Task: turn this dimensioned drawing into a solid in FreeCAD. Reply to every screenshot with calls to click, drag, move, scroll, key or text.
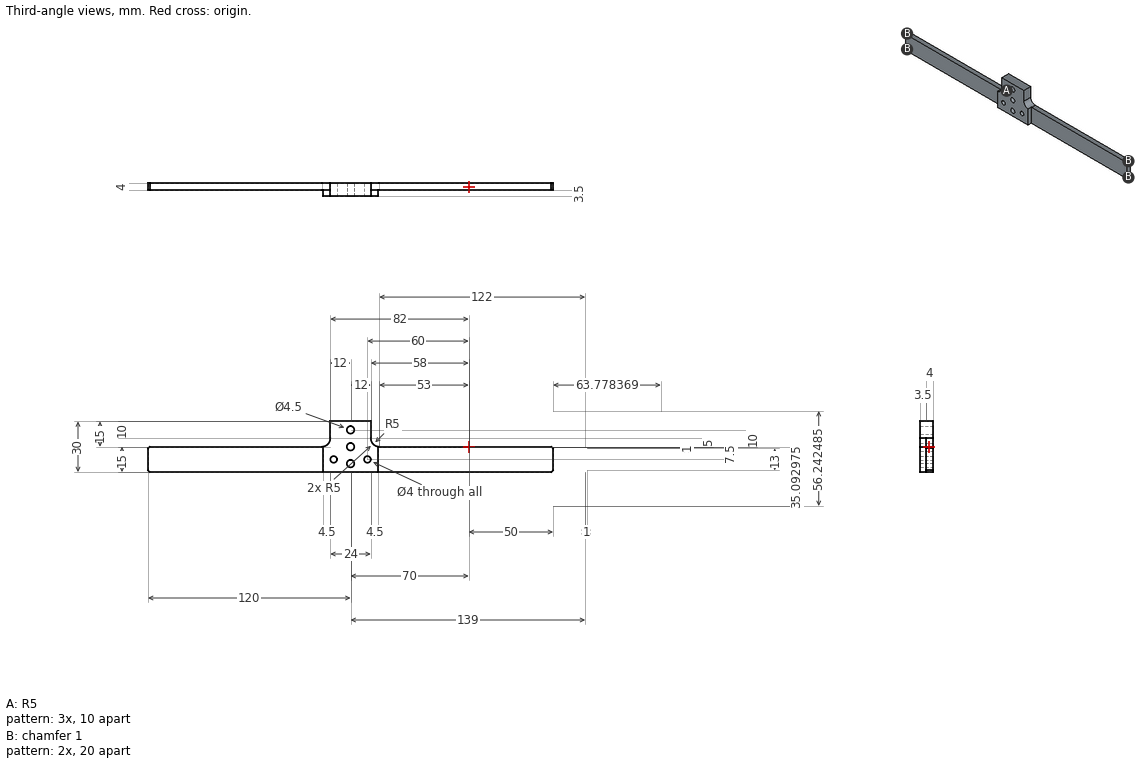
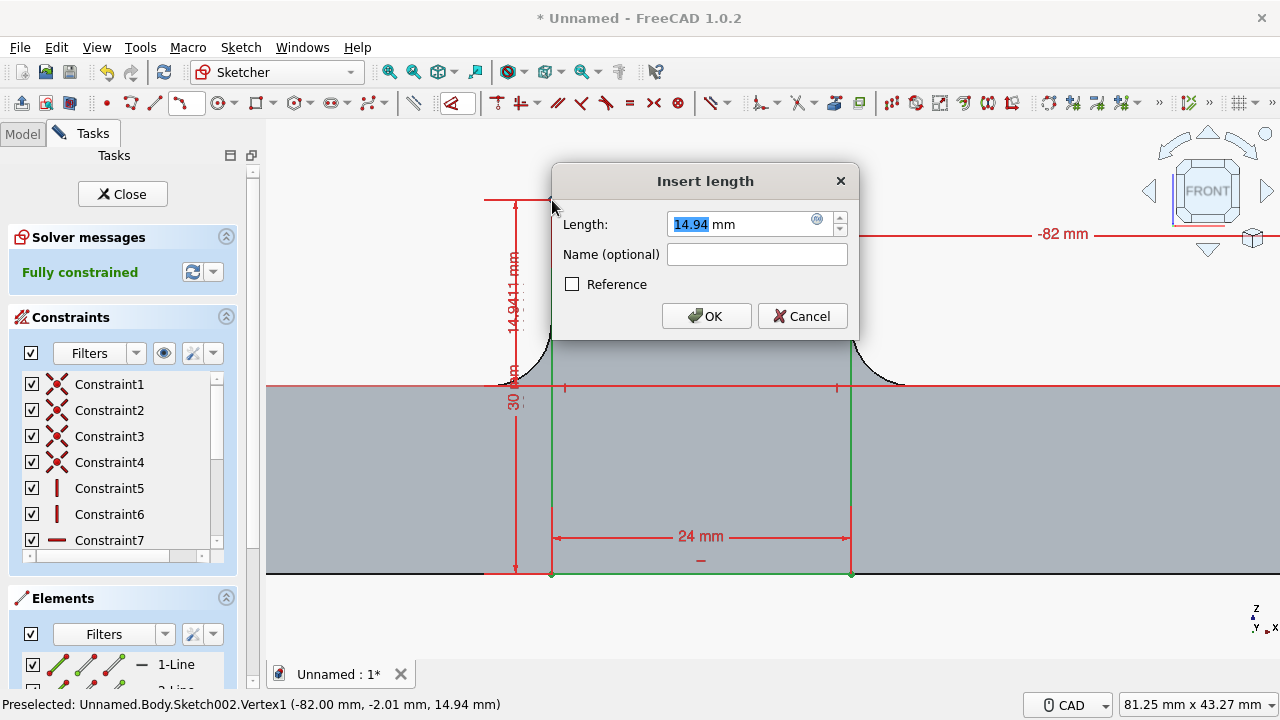
text(15)
key(Return)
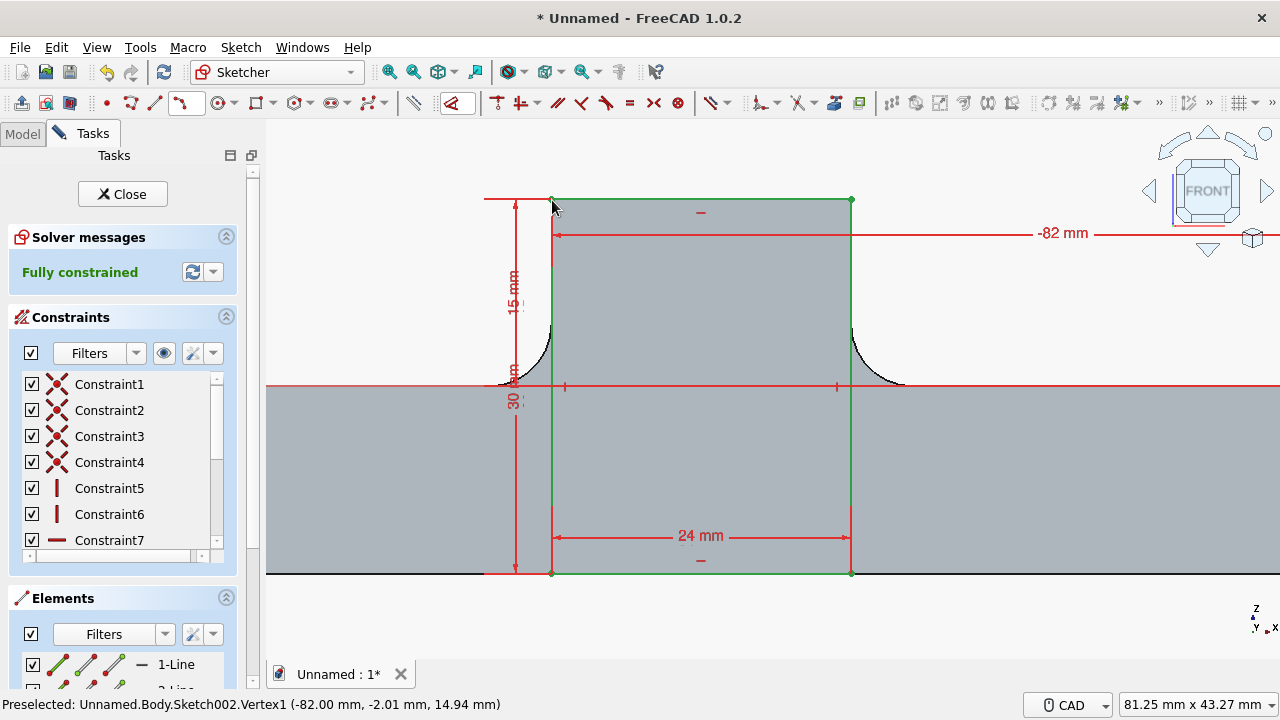
click(123, 194)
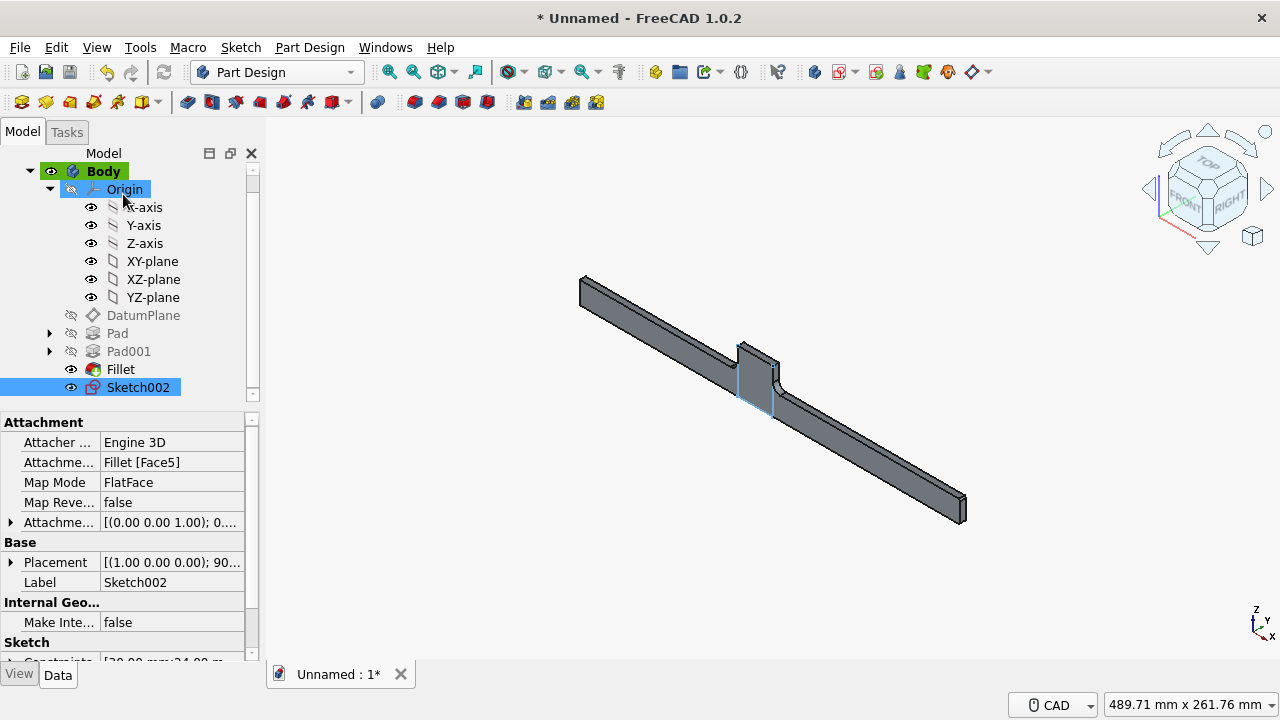
click(22, 102)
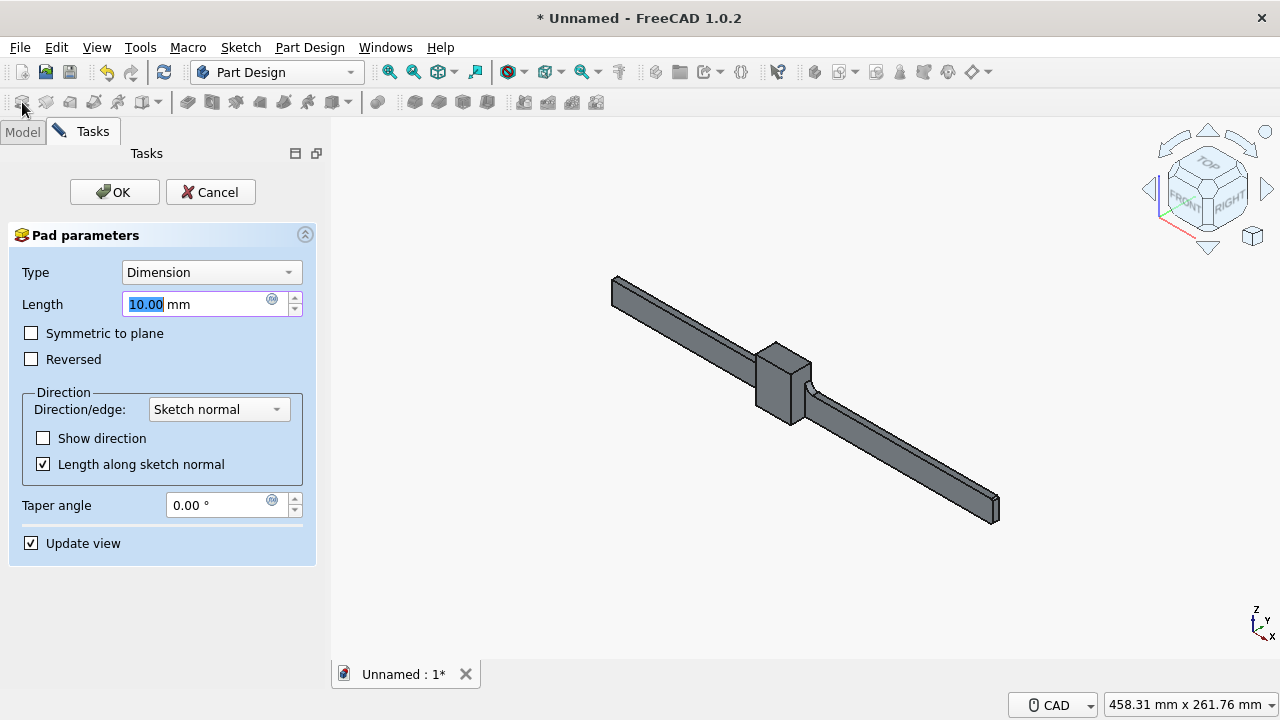
text(3.5)
key(Tab)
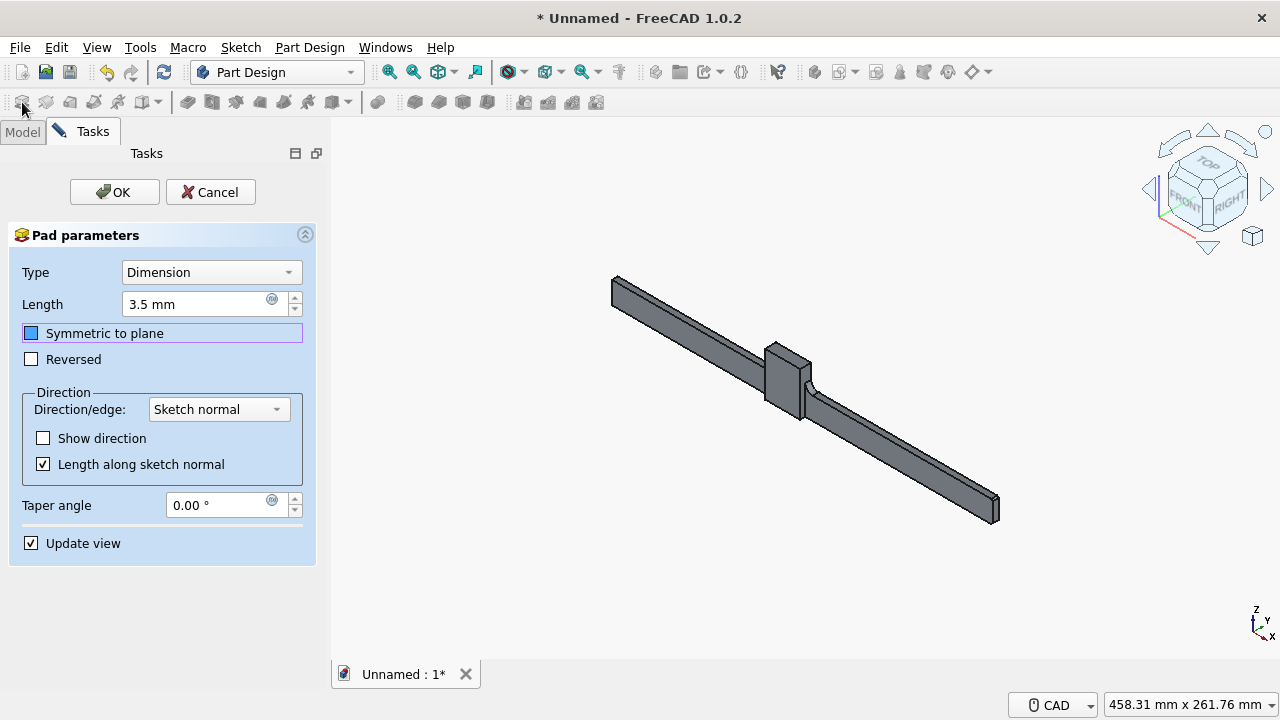
click(115, 192)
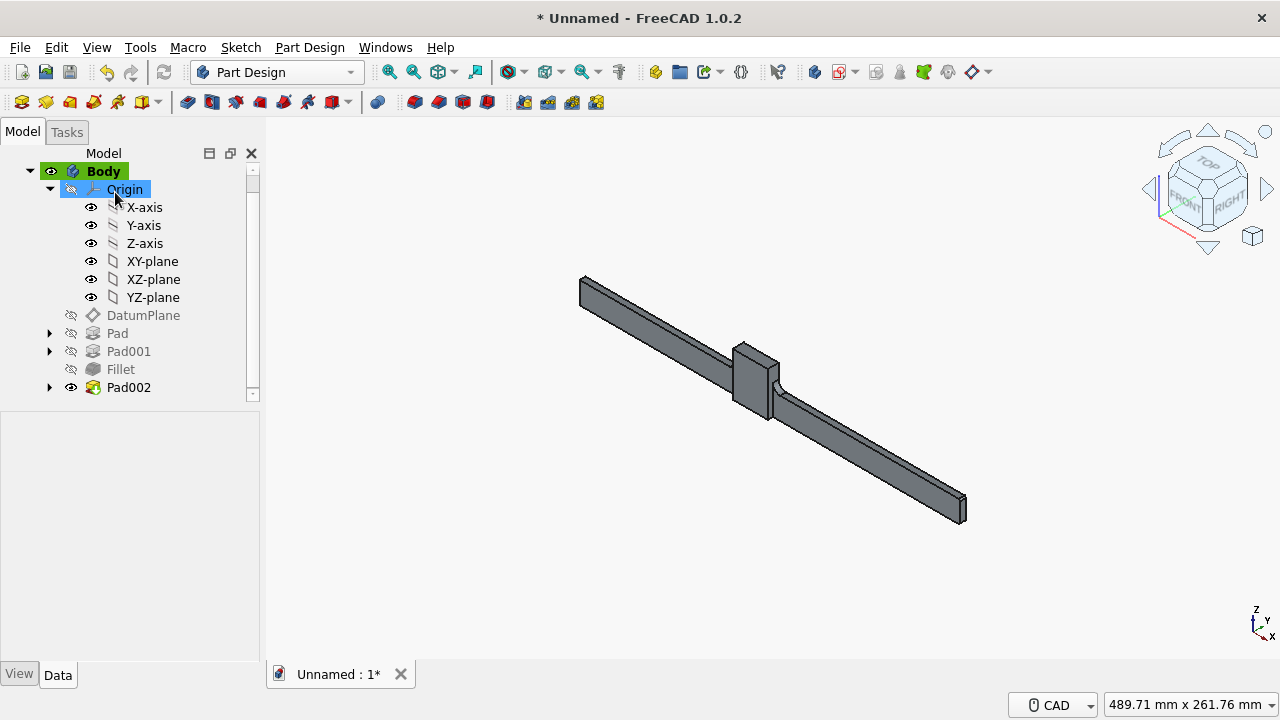
key(4)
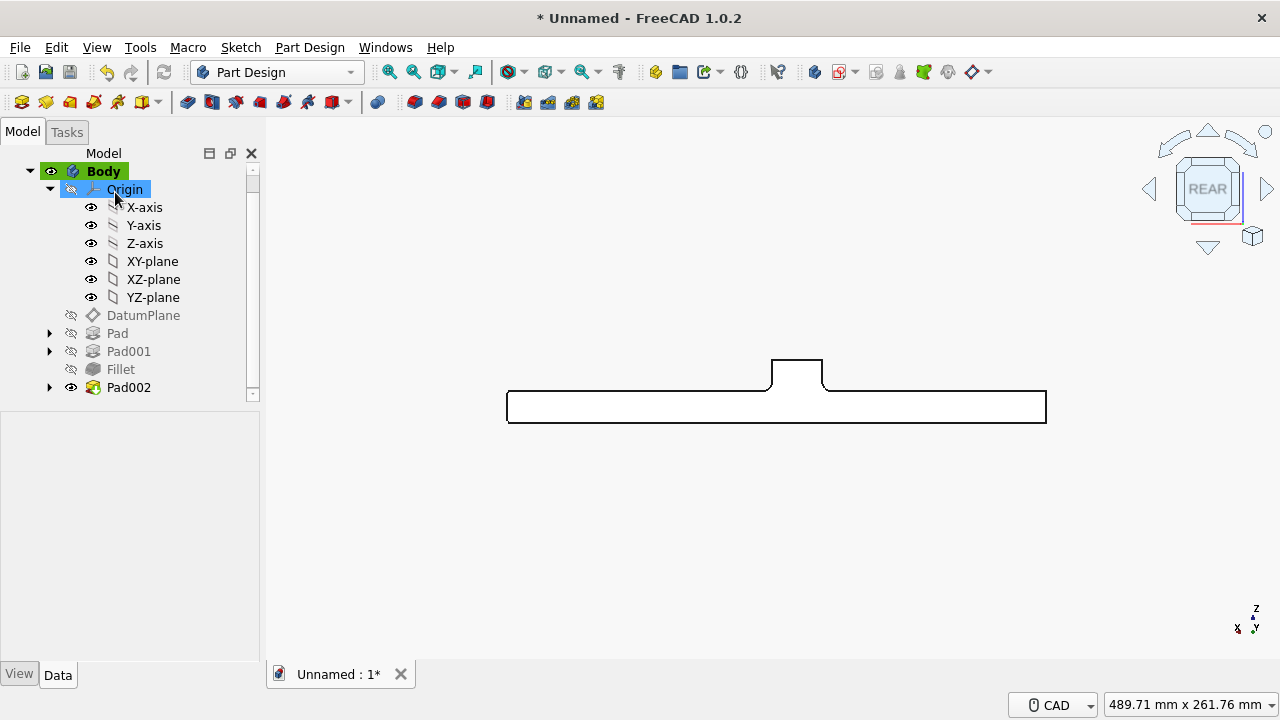
click(776, 399)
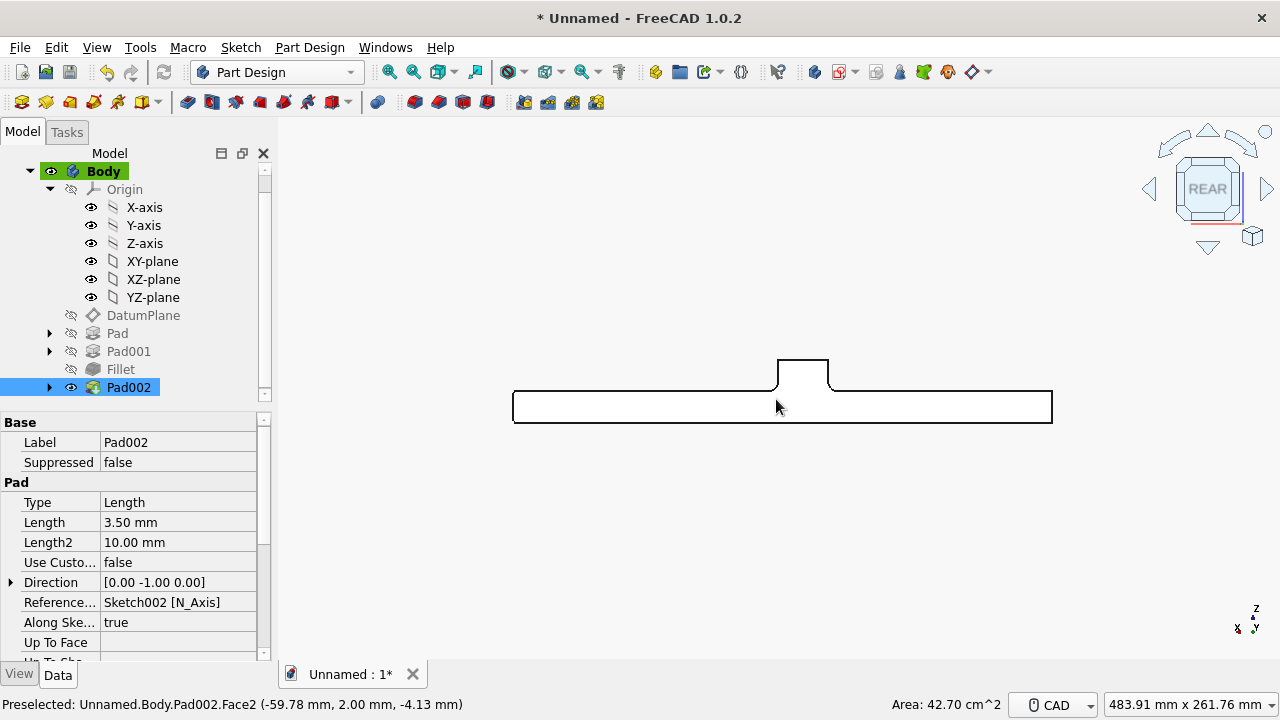
click(840, 72)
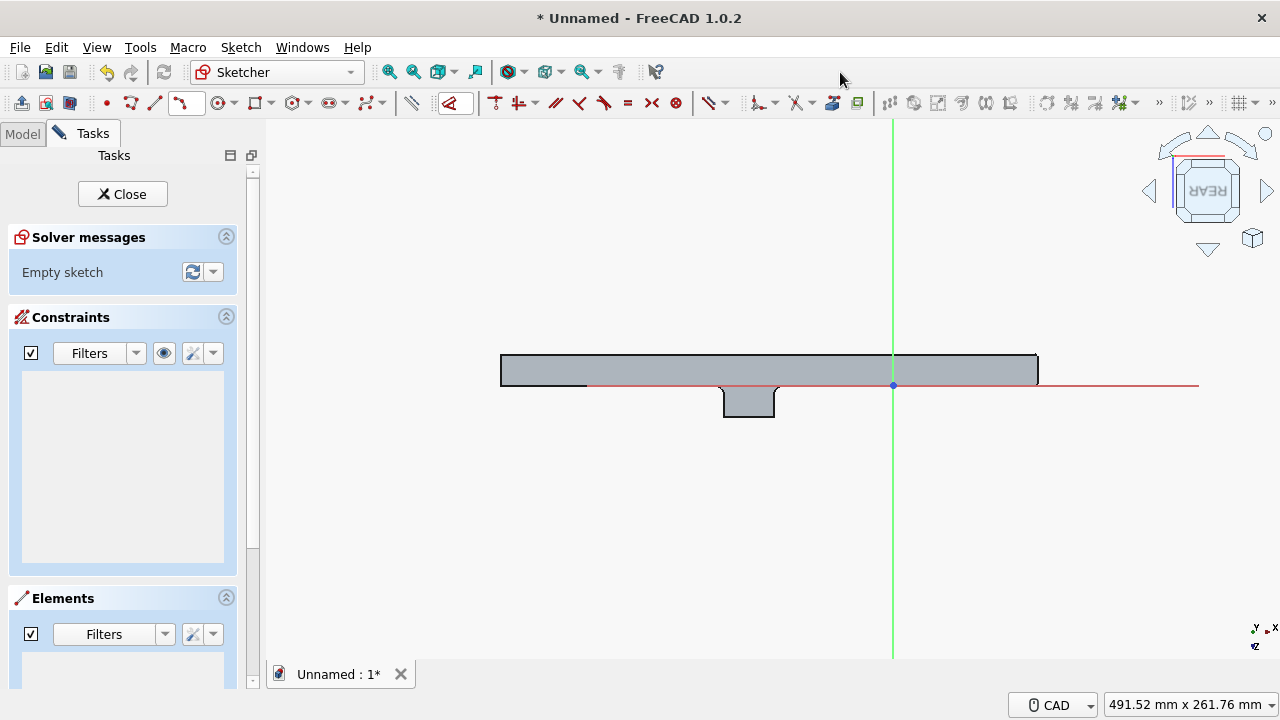
scroll(751, 407, up, 15)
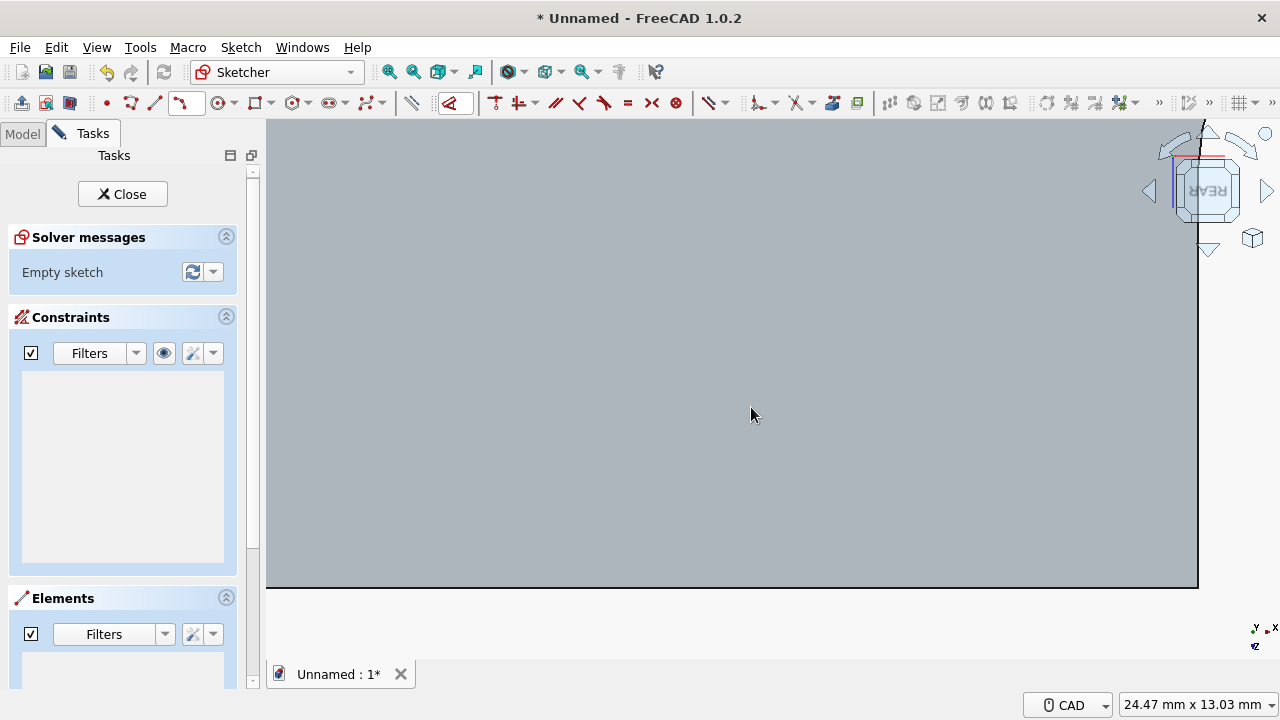
scroll(695, 370, up, 3)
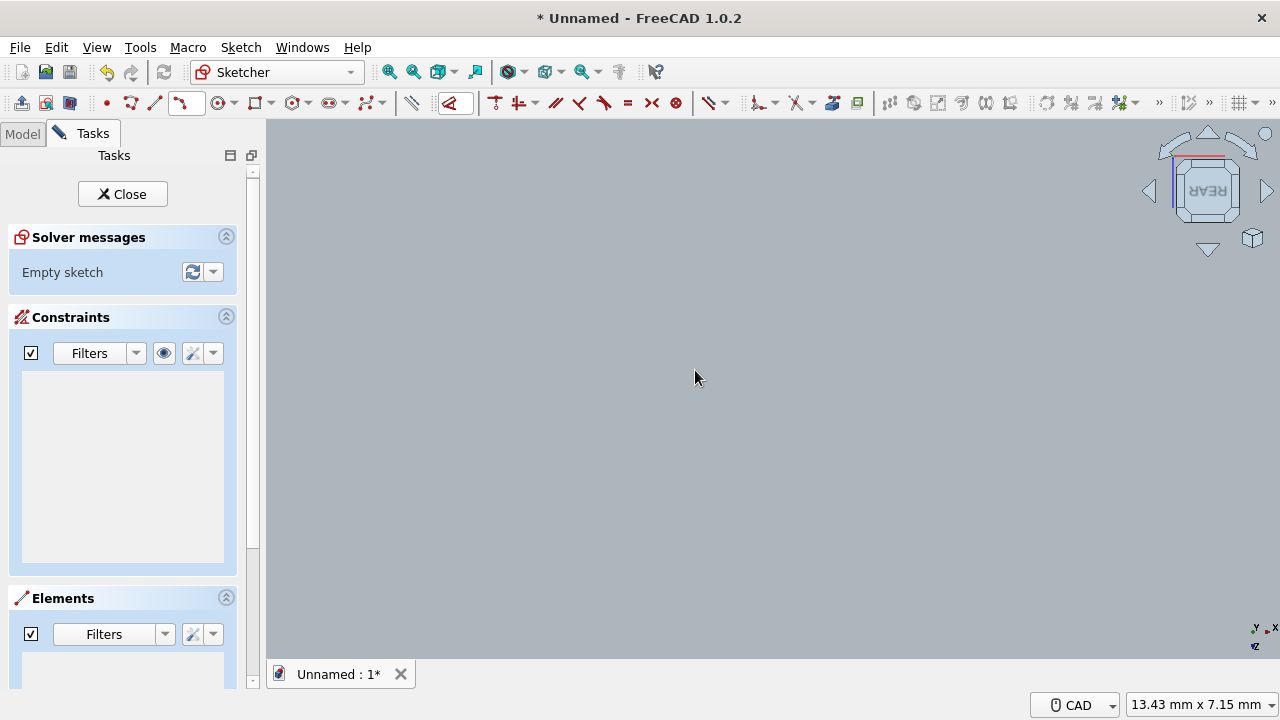
click(218, 104)